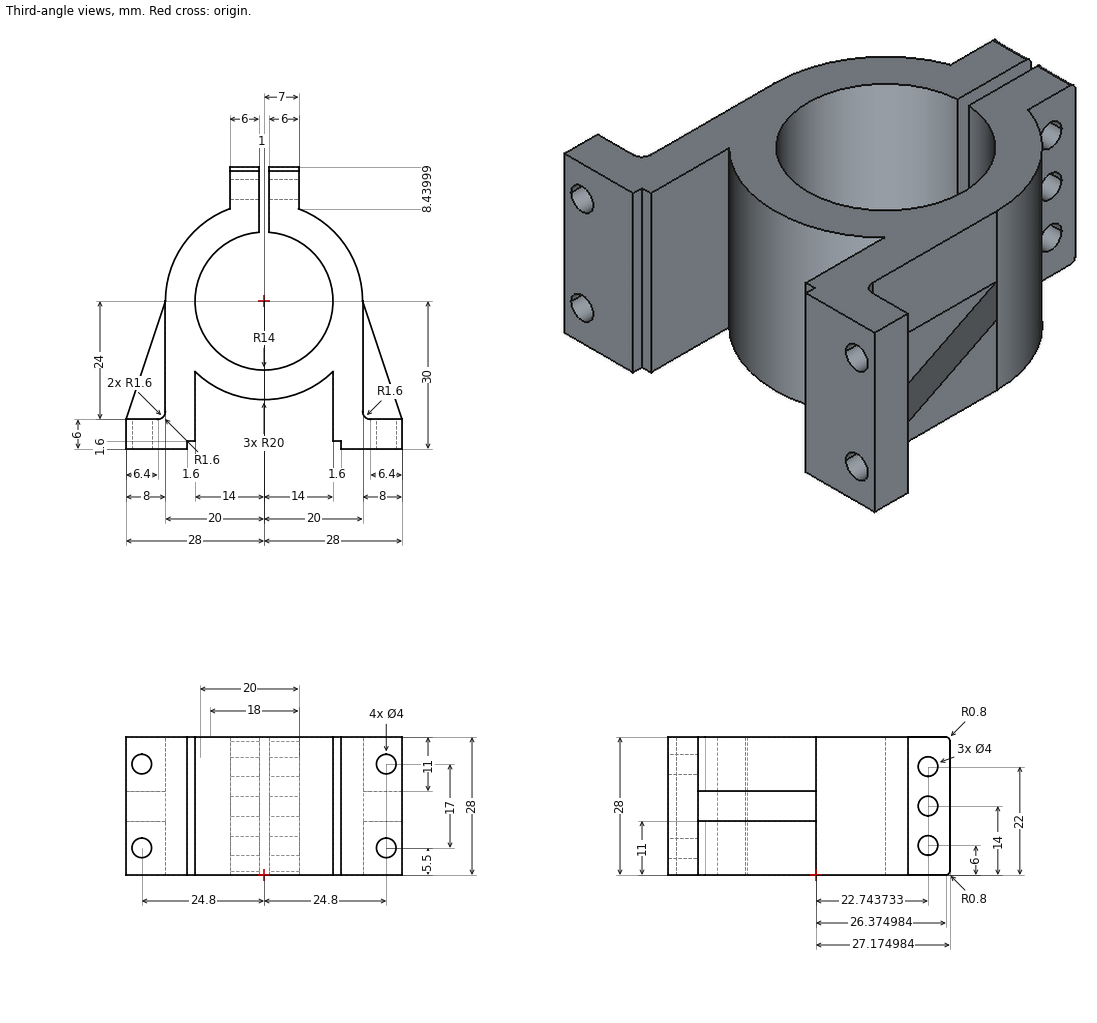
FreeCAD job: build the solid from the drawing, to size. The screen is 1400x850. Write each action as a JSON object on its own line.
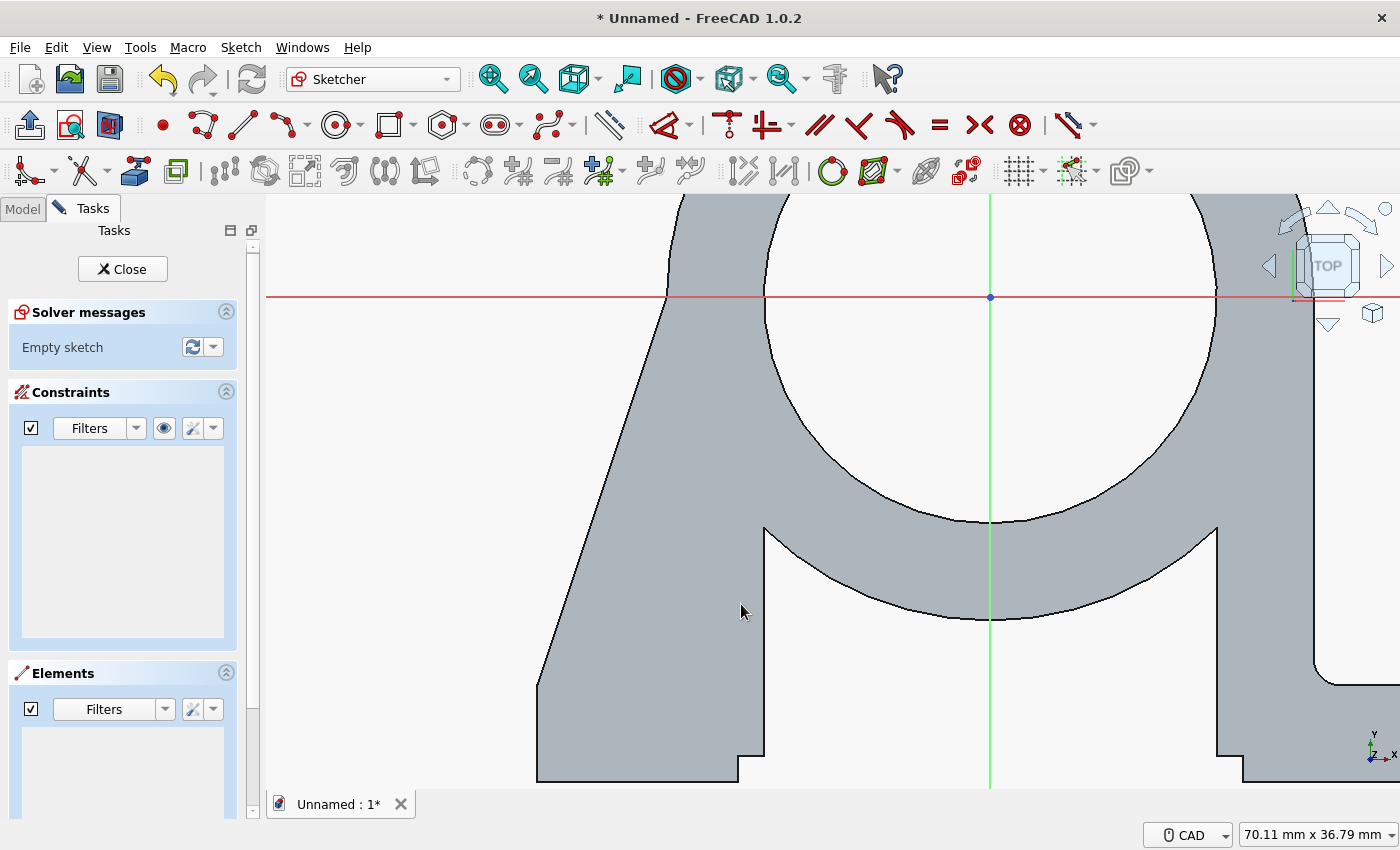
{"action": "left_click", "coordinate": [204, 126]}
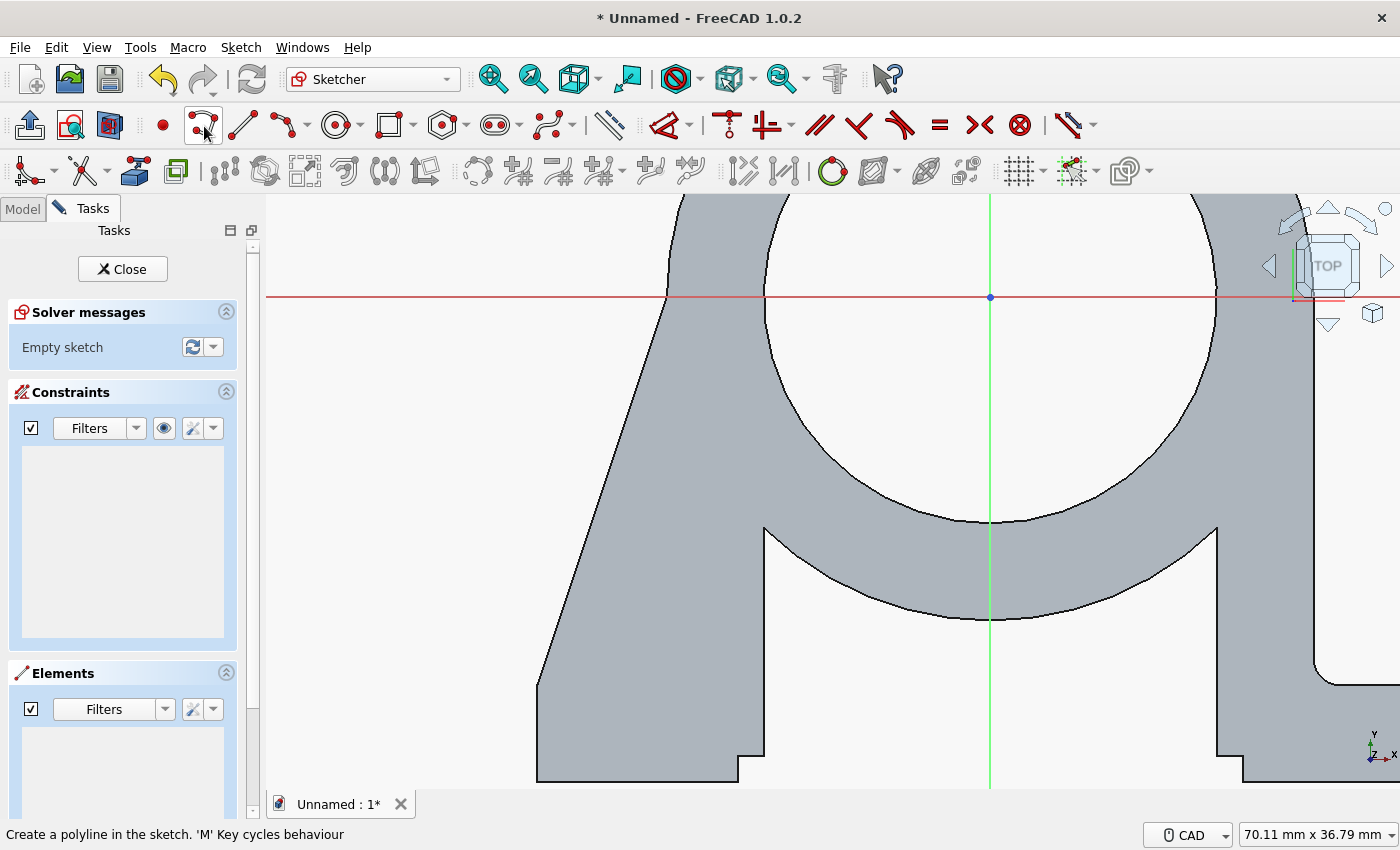
{"action": "left_click", "coordinate": [641, 685]}
{"action": "left_click", "coordinate": [537, 685]}
{"action": "left_click", "coordinate": [667, 297]}
{"action": "left_click", "coordinate": [667, 659]}
{"action": "right_click", "coordinate": [667, 659]}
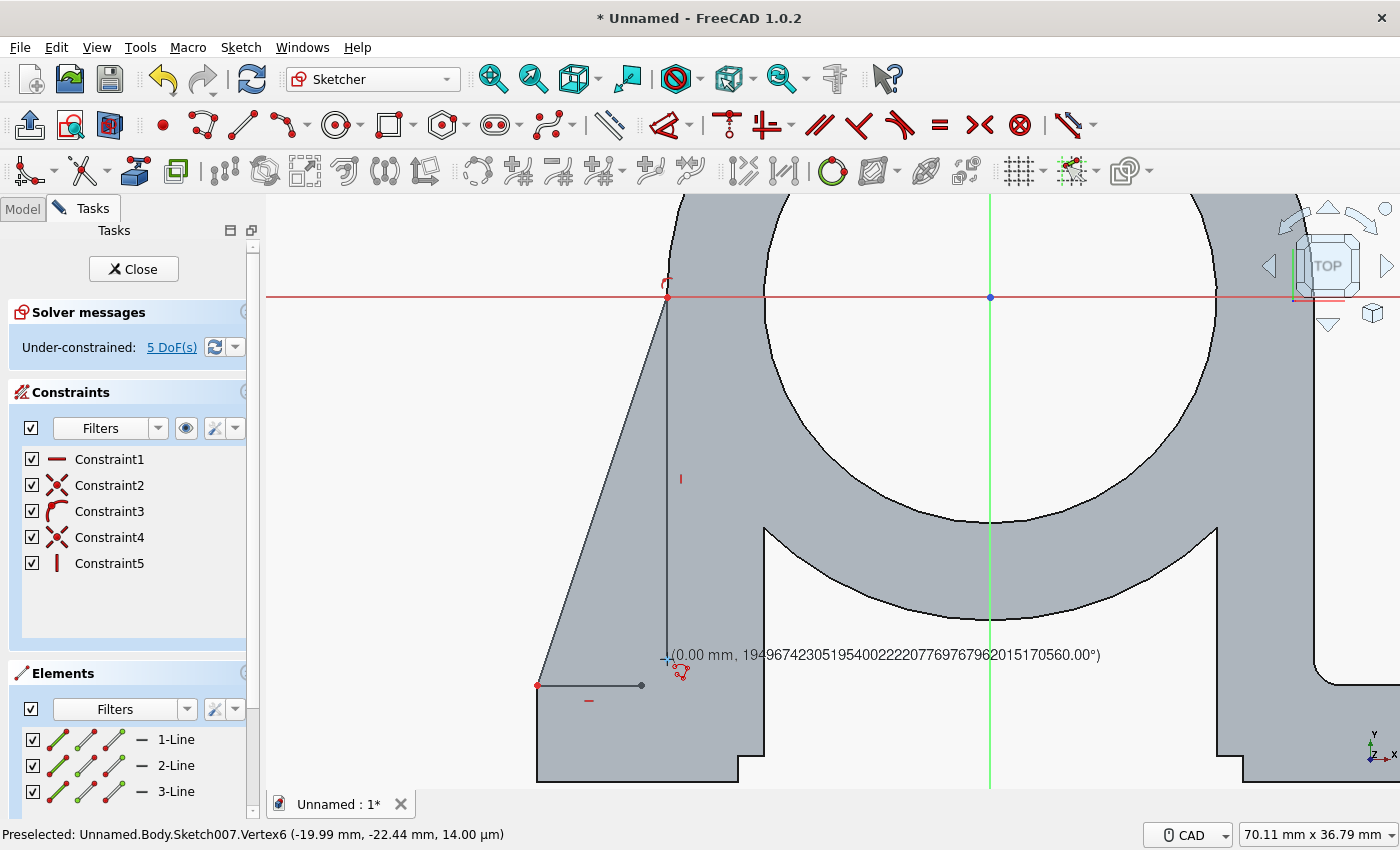
{"action": "left_click", "coordinate": [284, 126]}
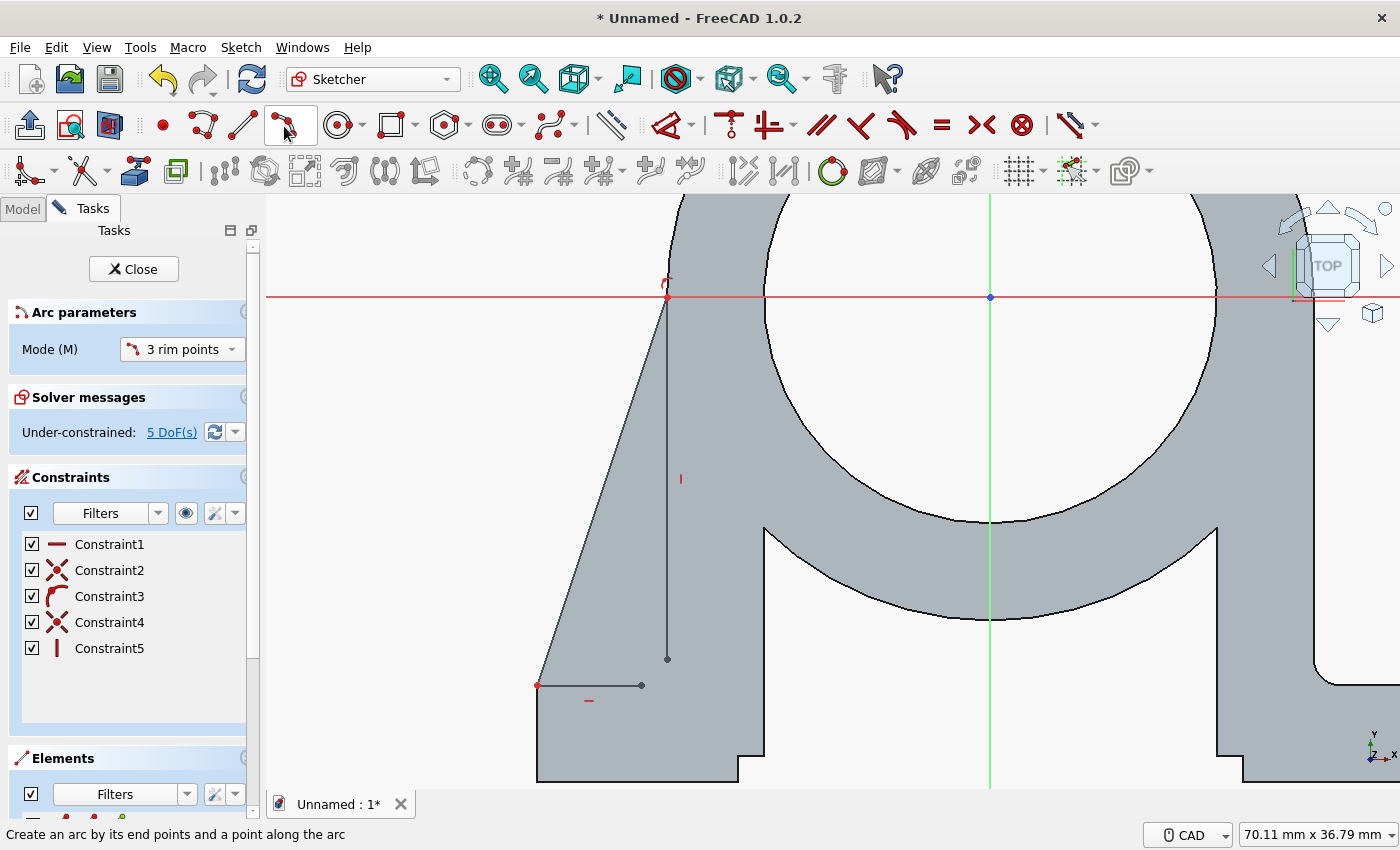
{"action": "left_click", "coordinate": [667, 660]}
{"action": "left_click", "coordinate": [641, 686]}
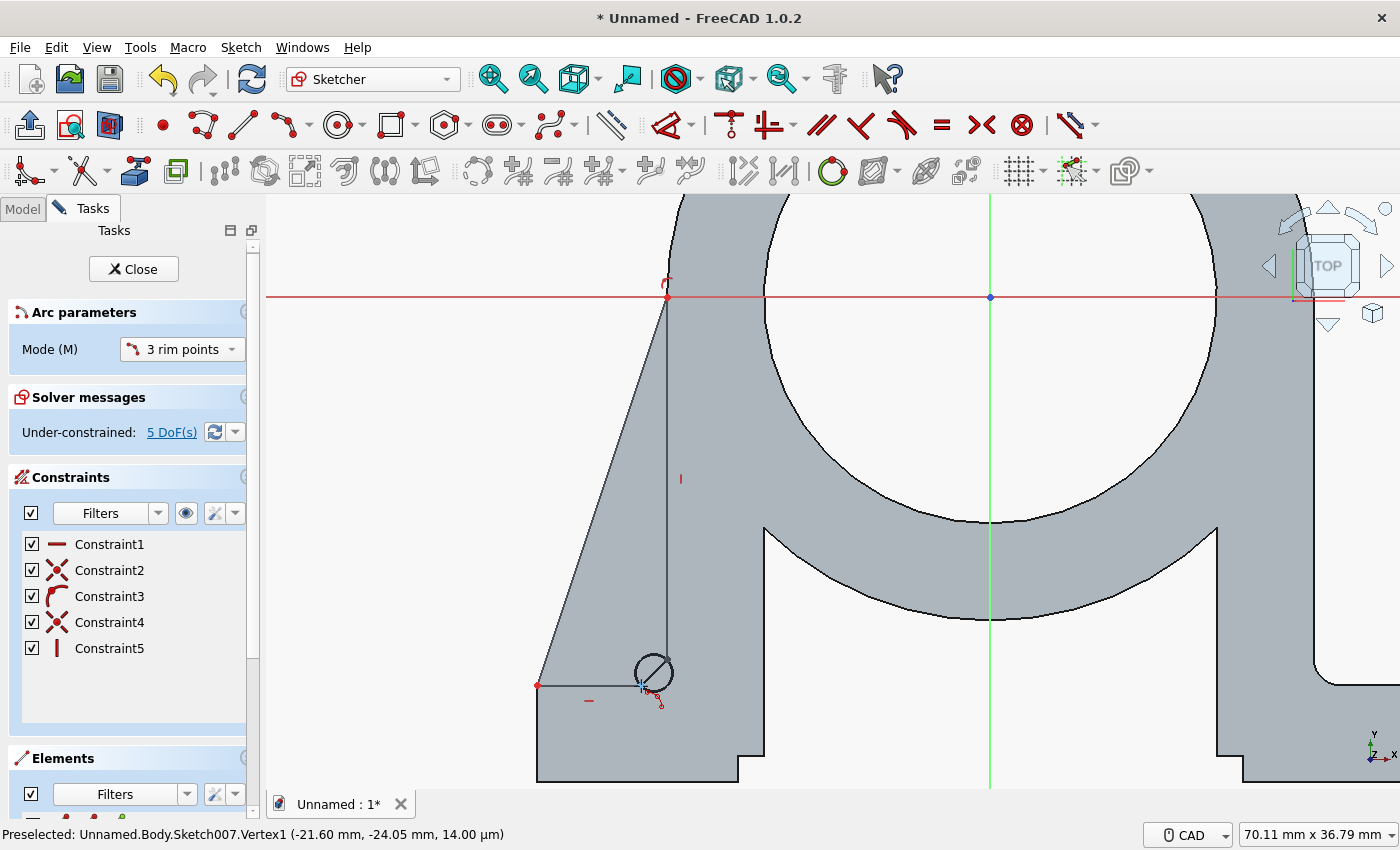
{"action": "scroll", "coordinate": [659, 678], "scroll_direction": "up", "scroll_amount": 4}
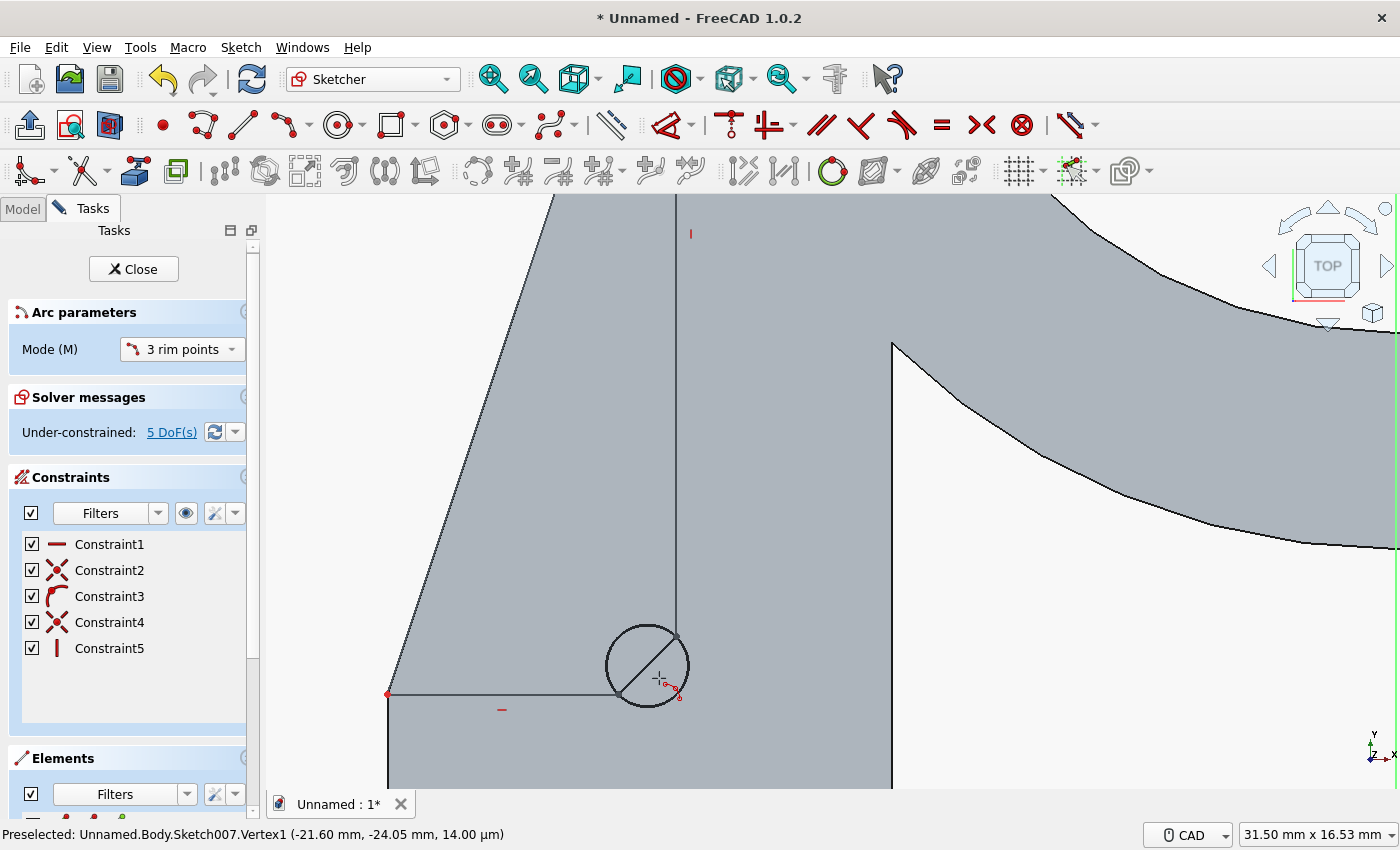
{"action": "left_click", "coordinate": [659, 676]}
{"action": "key", "text": "Escape"}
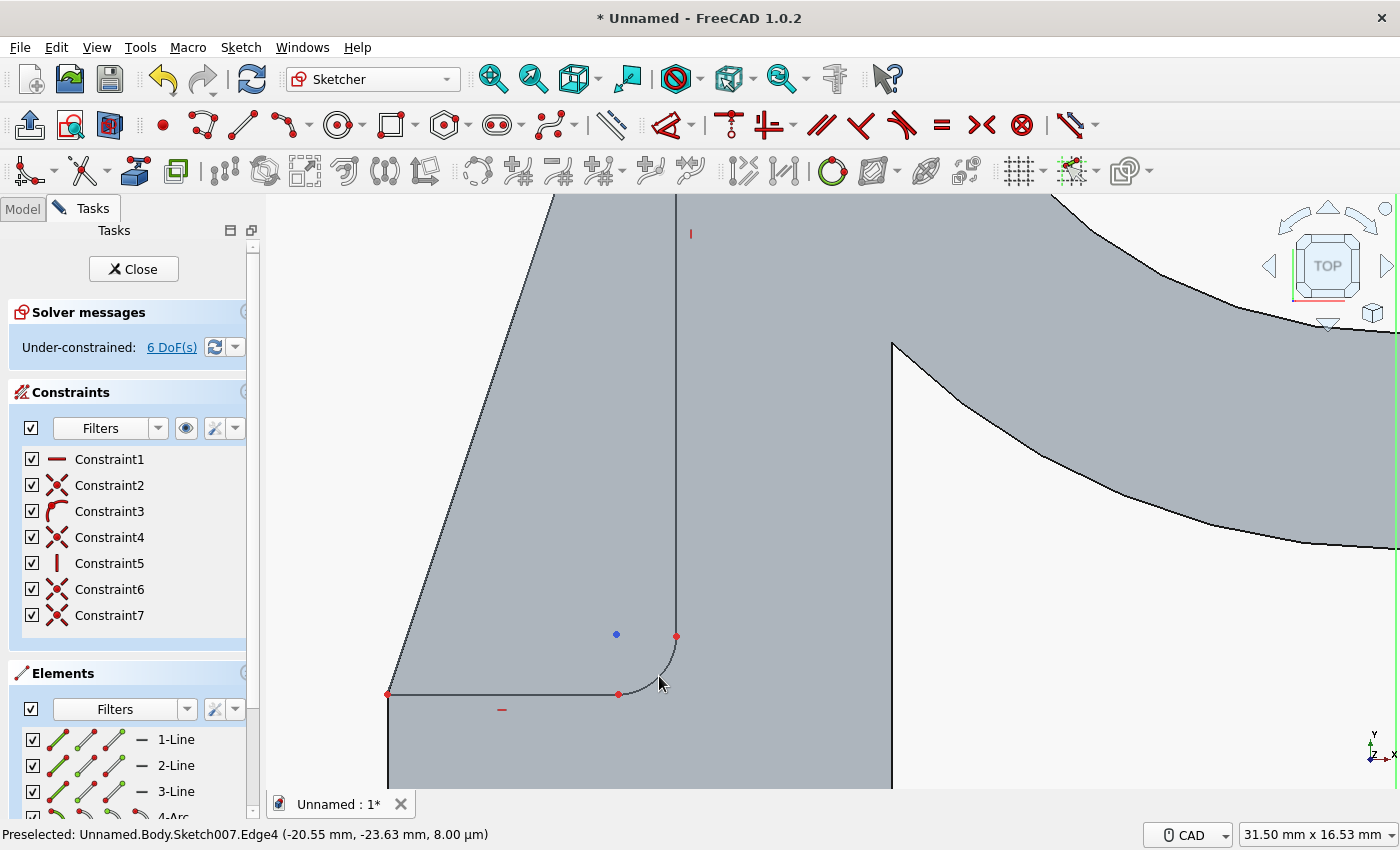
{"action": "left_click", "coordinate": [549, 695]}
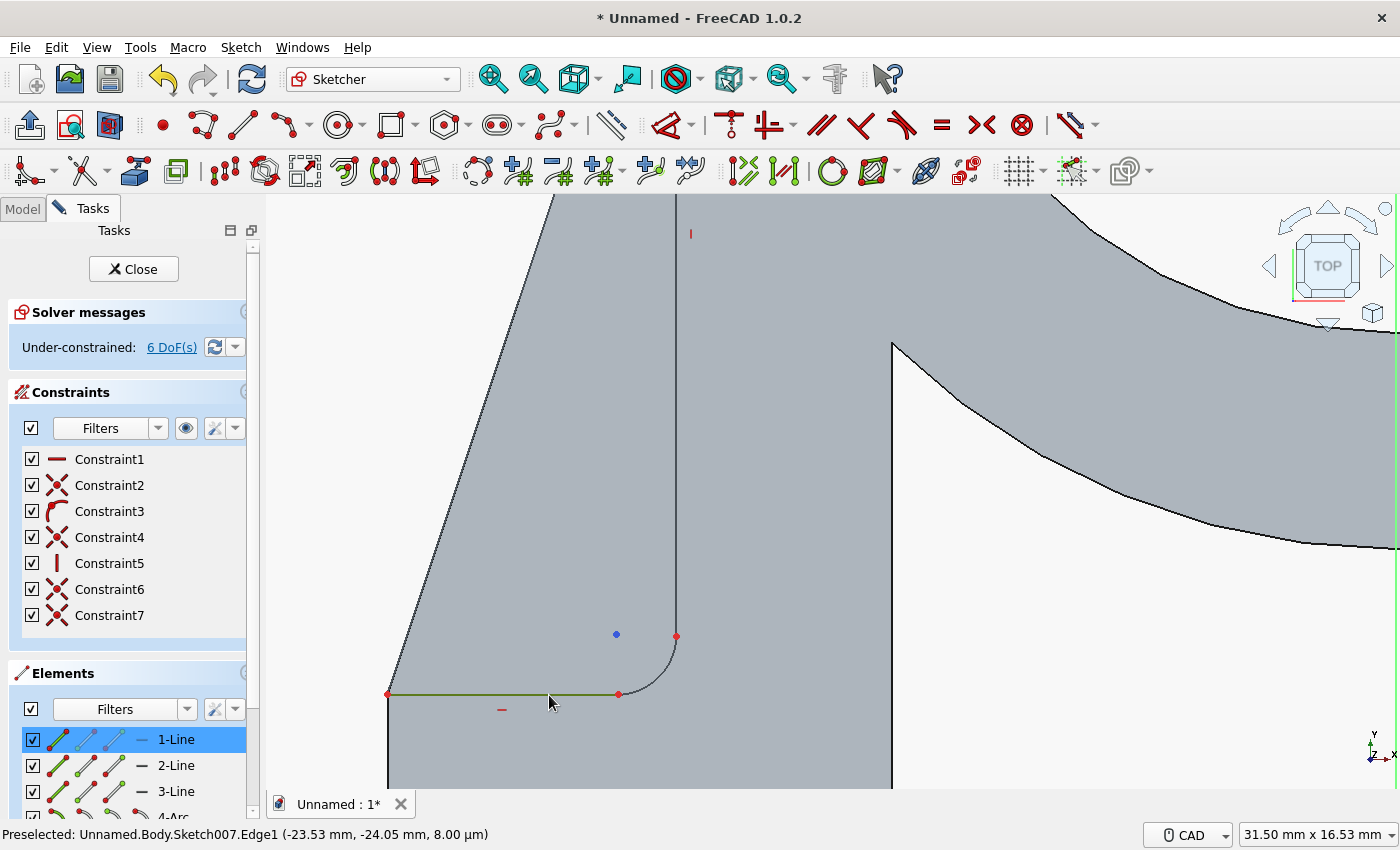
{"action": "left_click", "coordinate": [644, 688]}